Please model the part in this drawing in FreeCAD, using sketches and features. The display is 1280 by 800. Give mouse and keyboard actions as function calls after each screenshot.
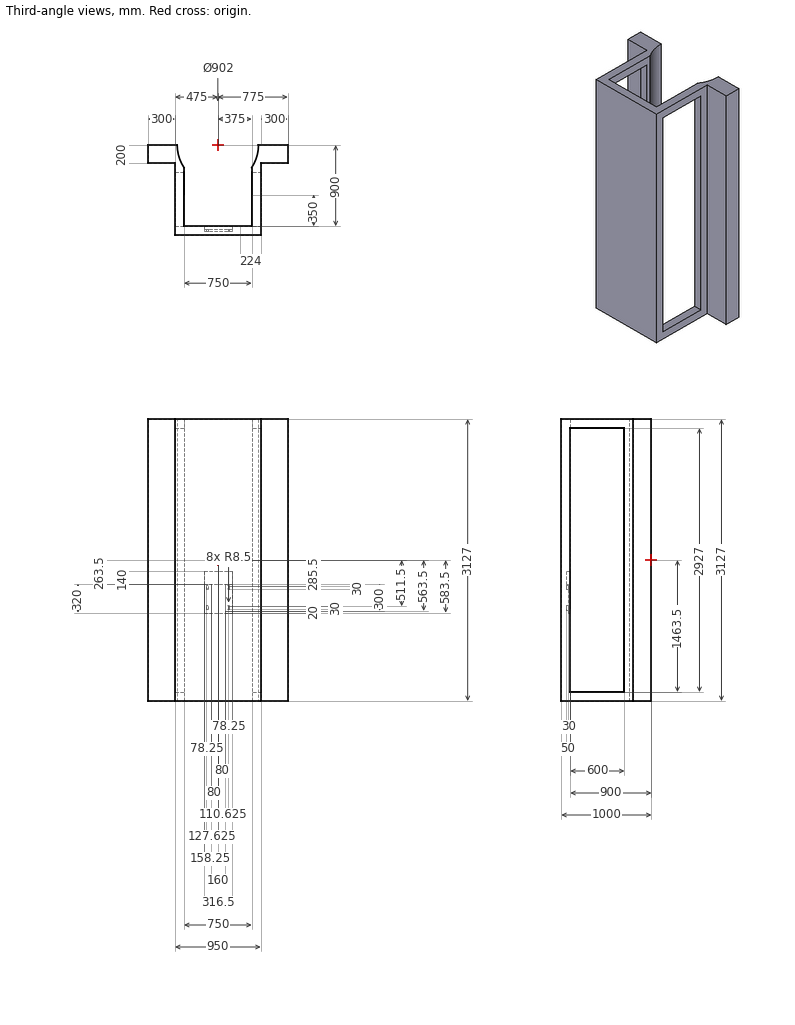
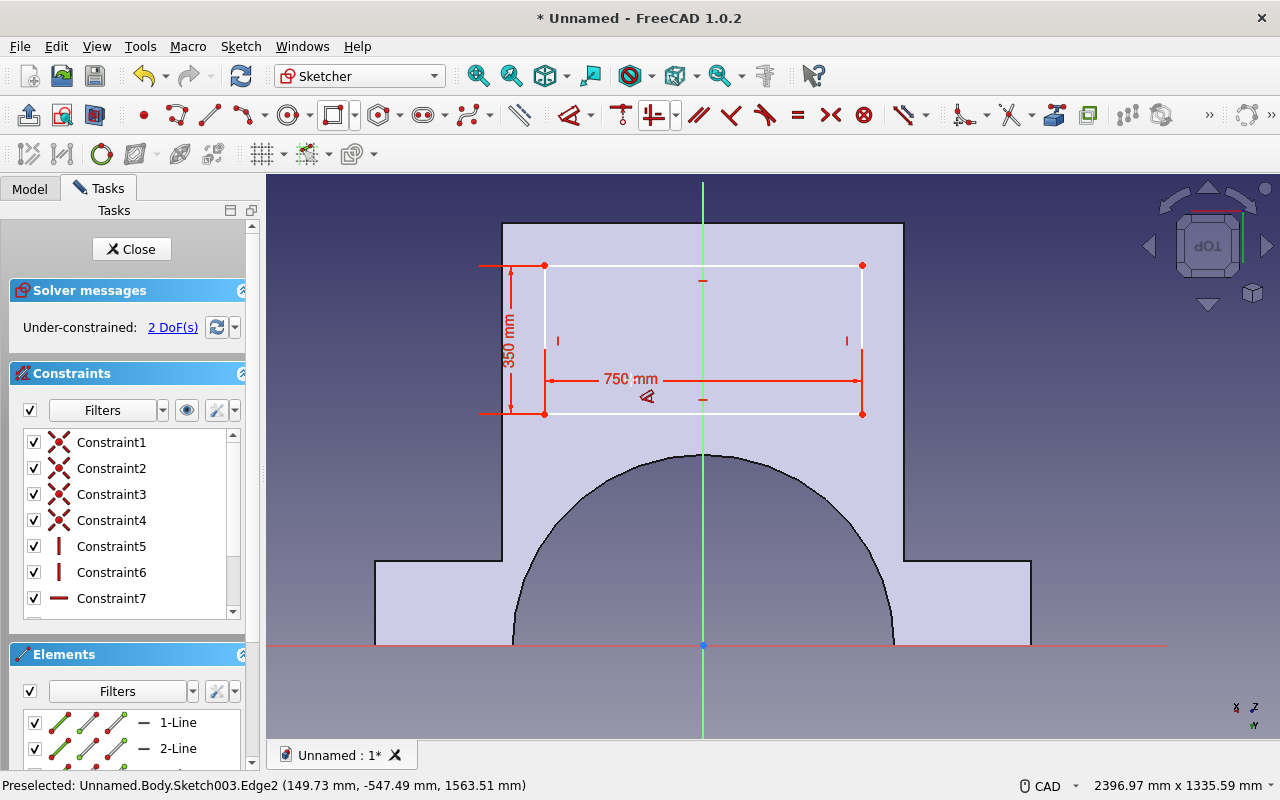
click(545, 266)
click(624, 680)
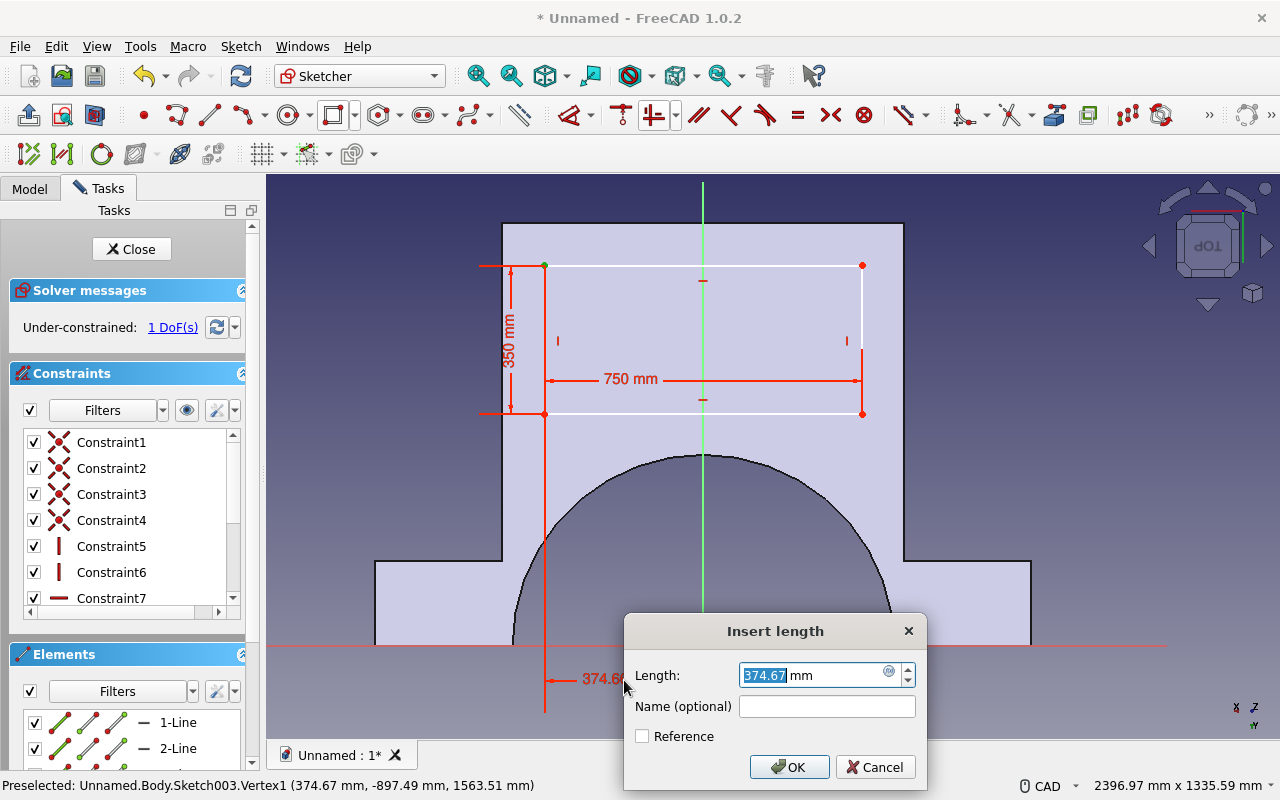
text(375)
key(Return)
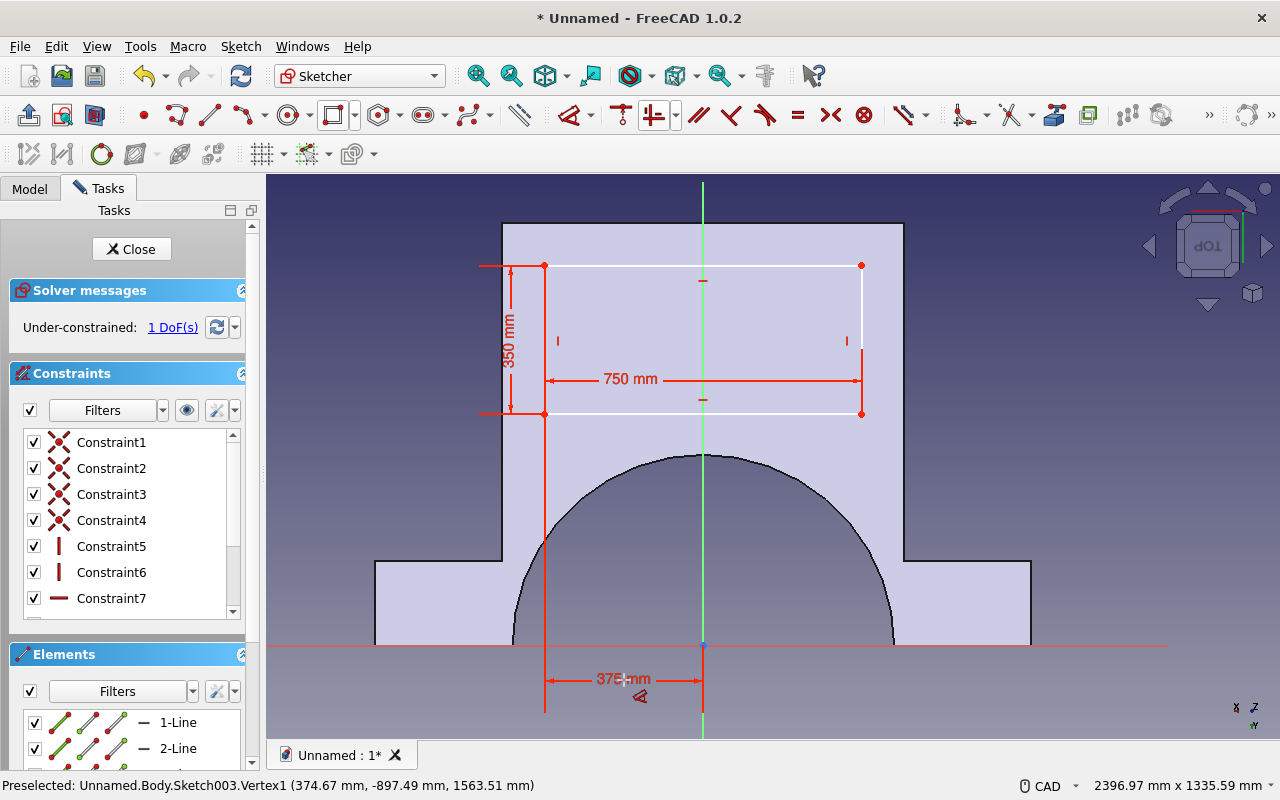
click(545, 266)
click(511, 456)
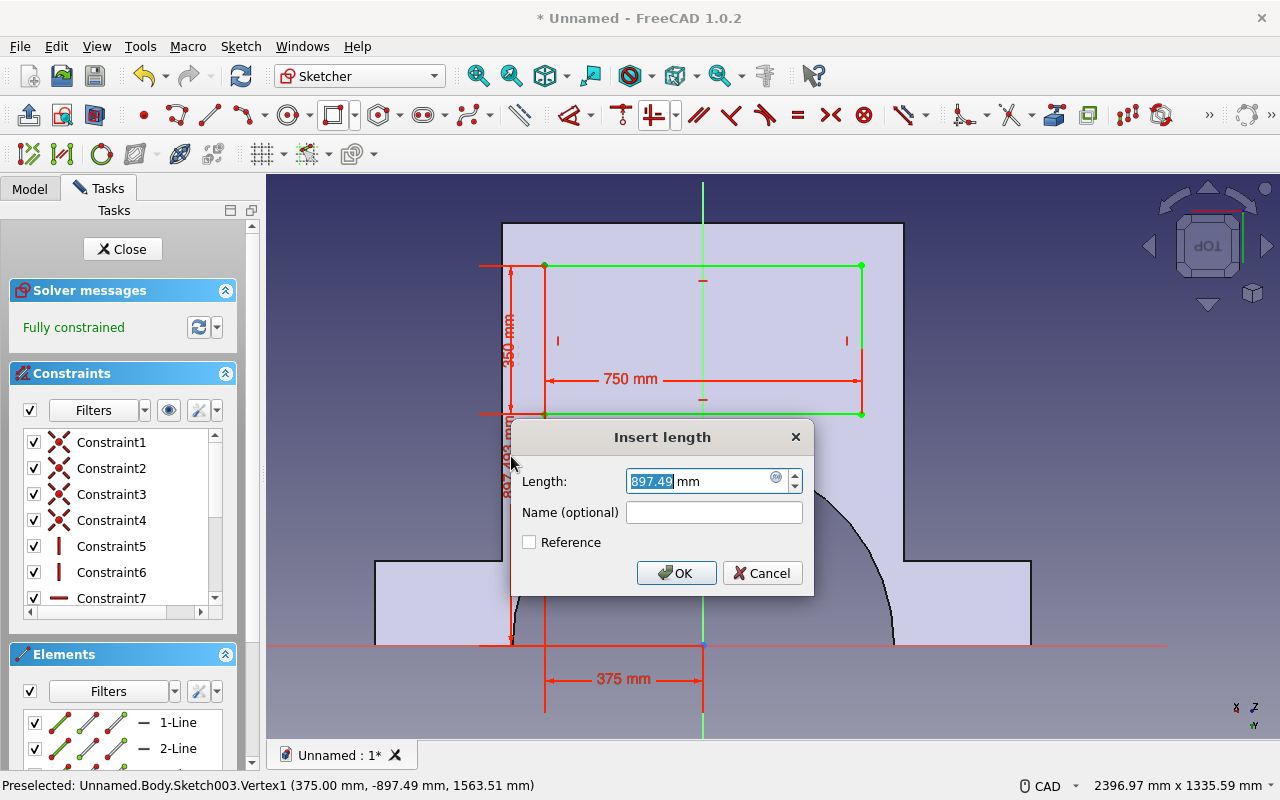
text(900)
key(Return)
key(Escape)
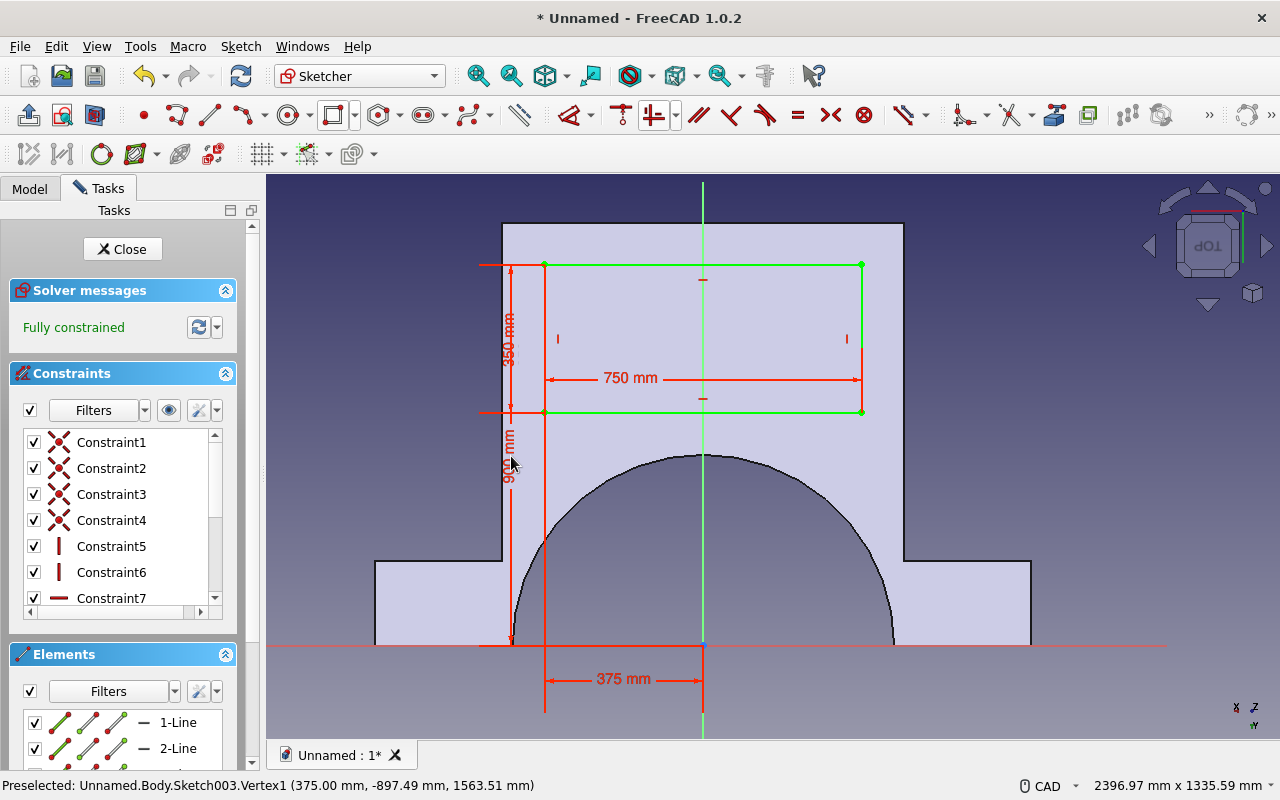
click(123, 249)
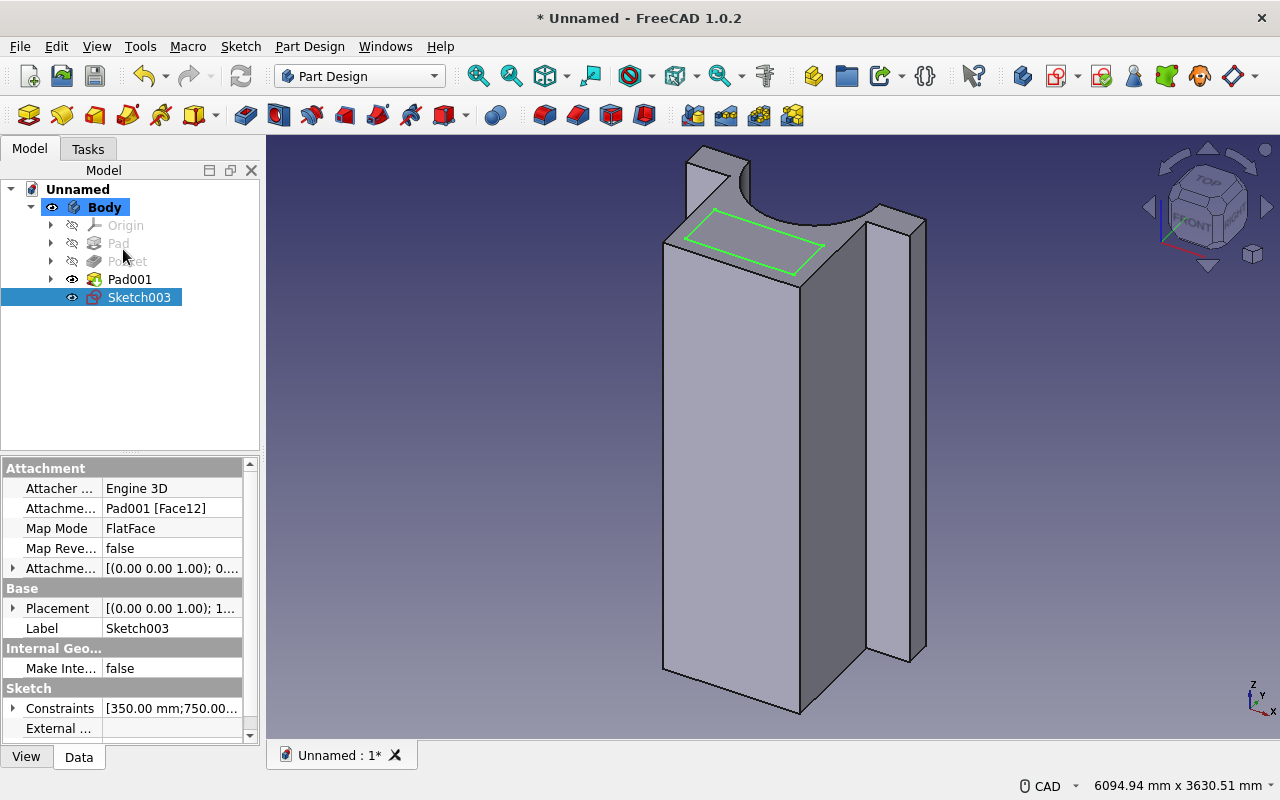
click(246, 116)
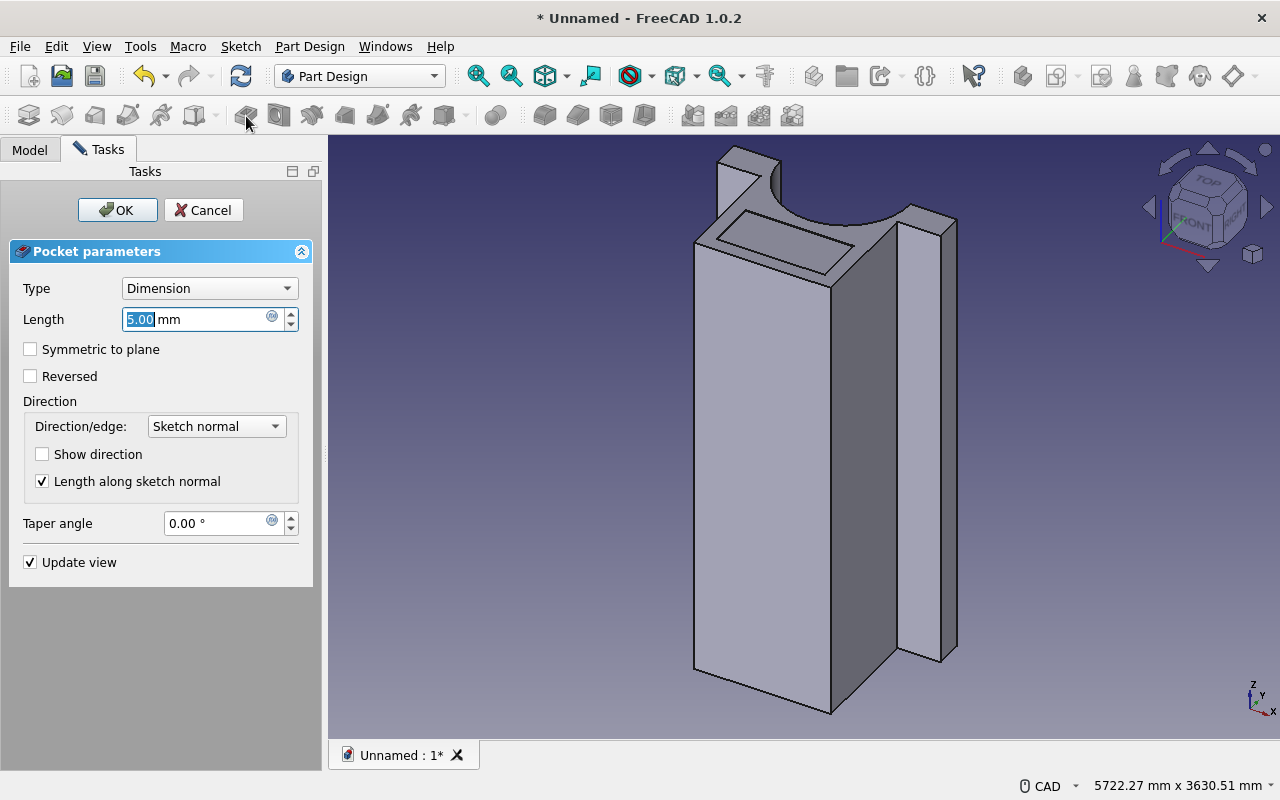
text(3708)
key(Tab)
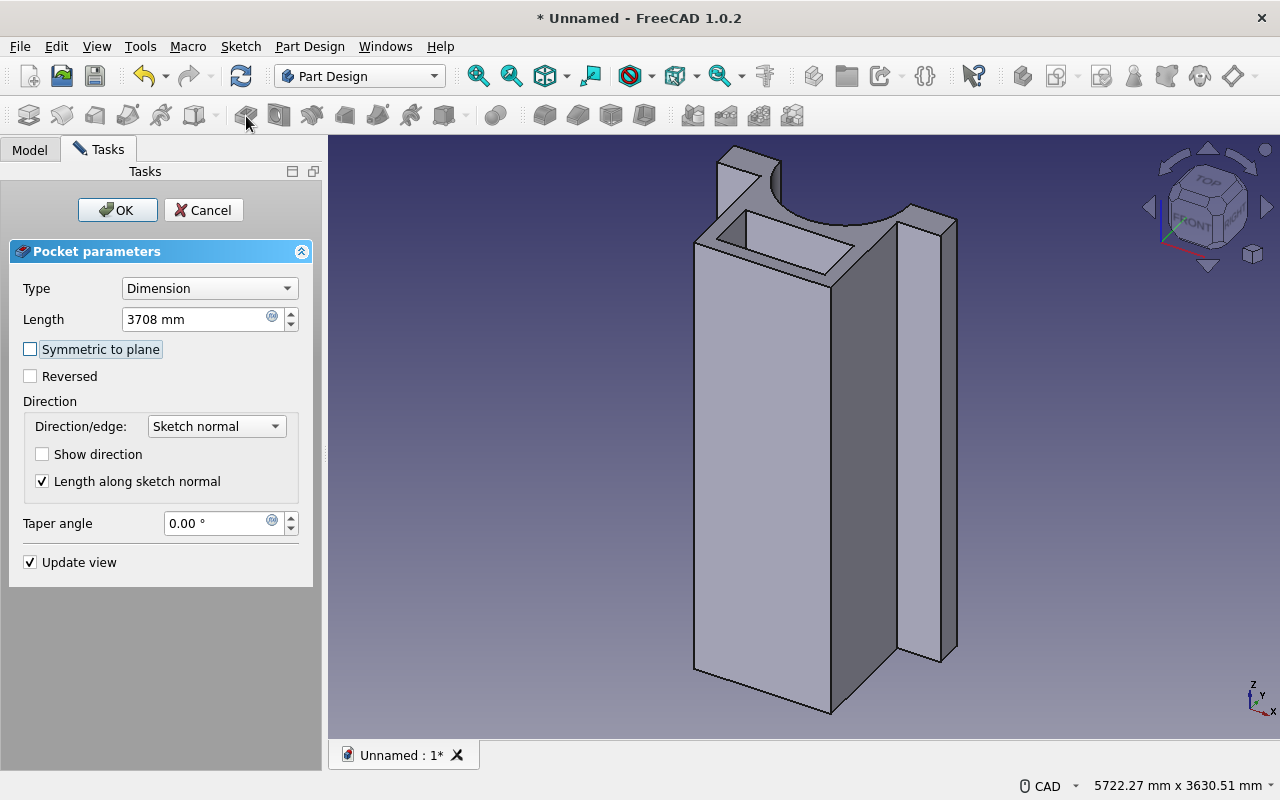
click(118, 210)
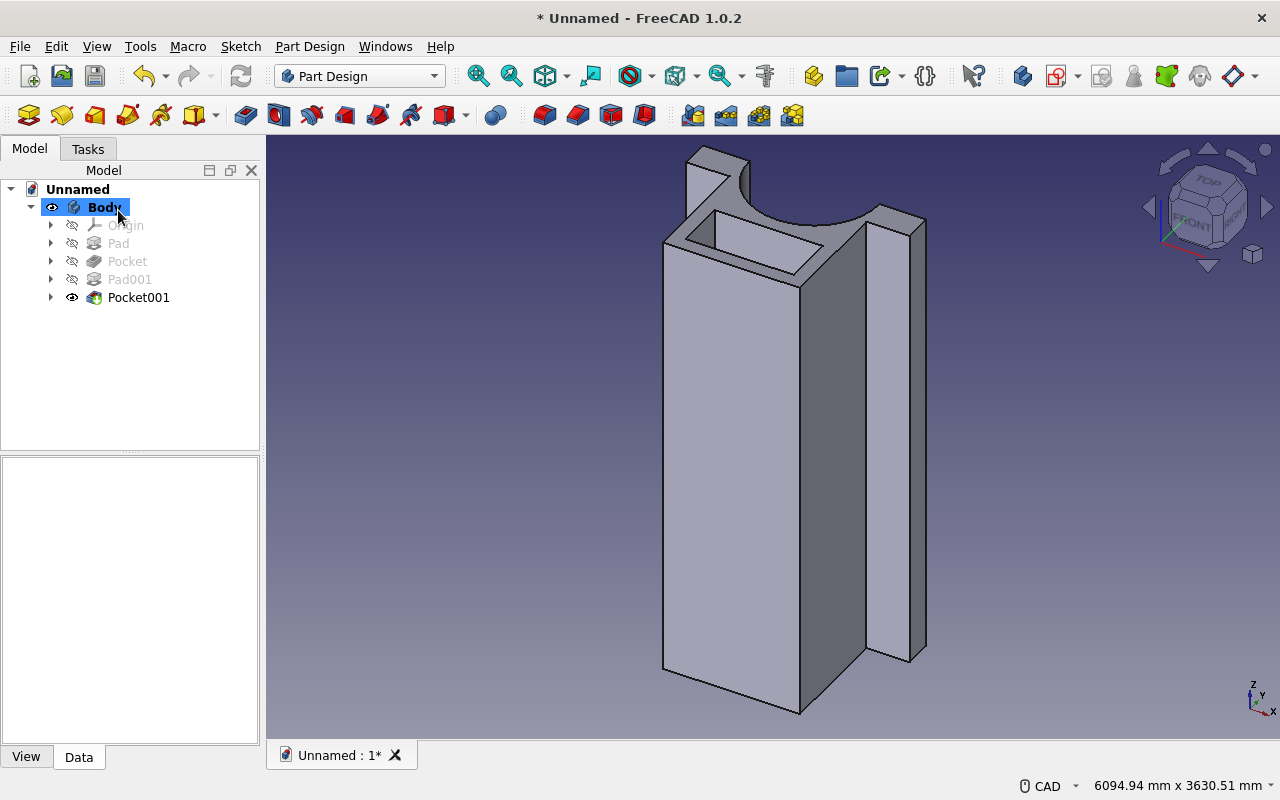
click(51, 225)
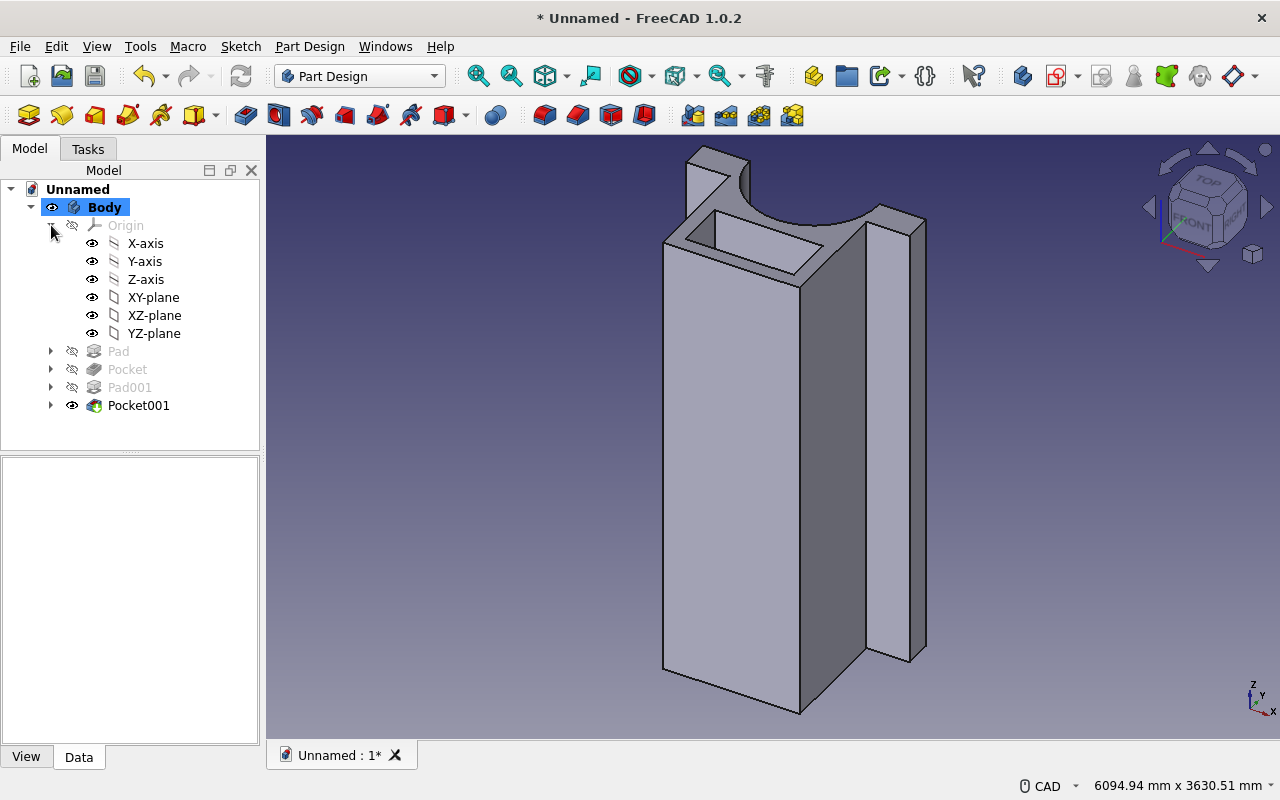
click(137, 315)